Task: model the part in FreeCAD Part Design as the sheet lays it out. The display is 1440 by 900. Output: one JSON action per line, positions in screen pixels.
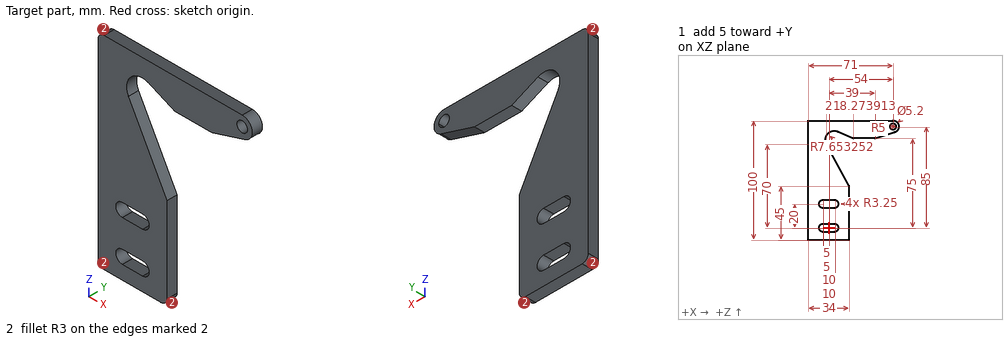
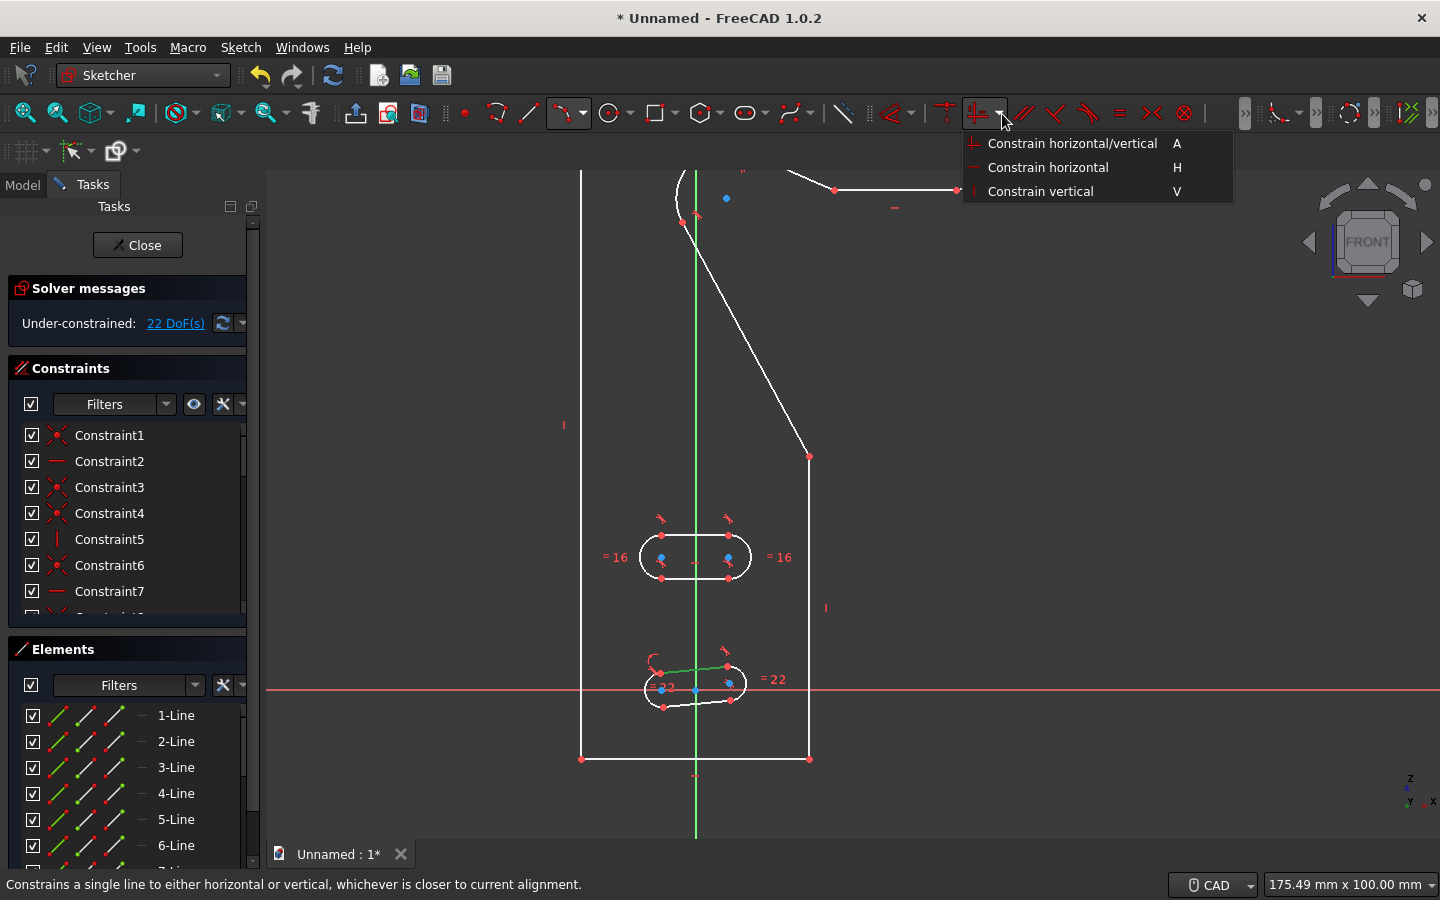
{"action": "left_click", "coordinate": [1098, 167]}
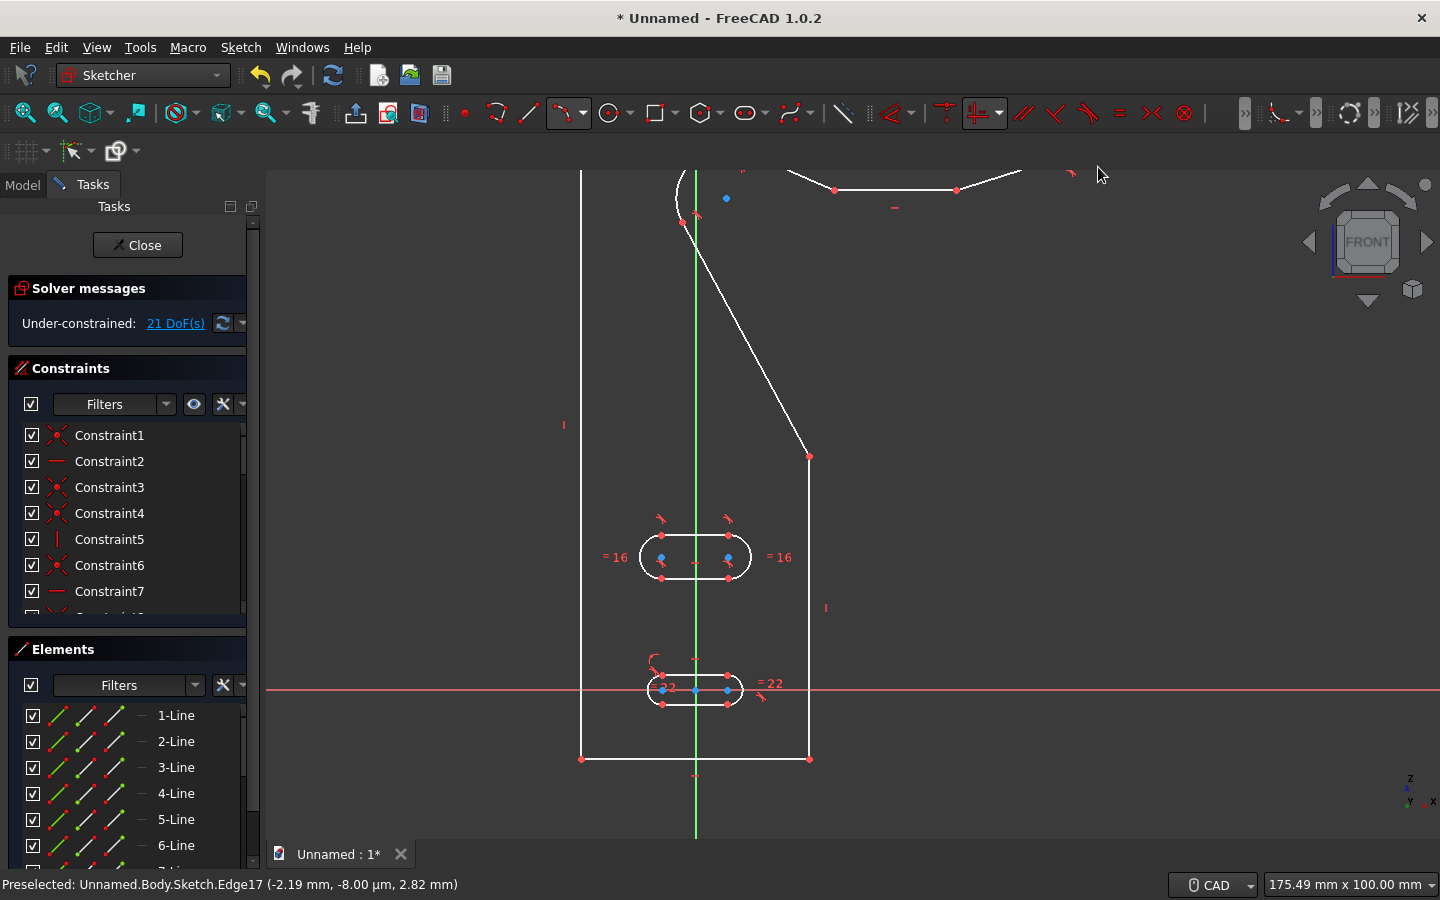
{"action": "left_click", "coordinate": [644, 544]}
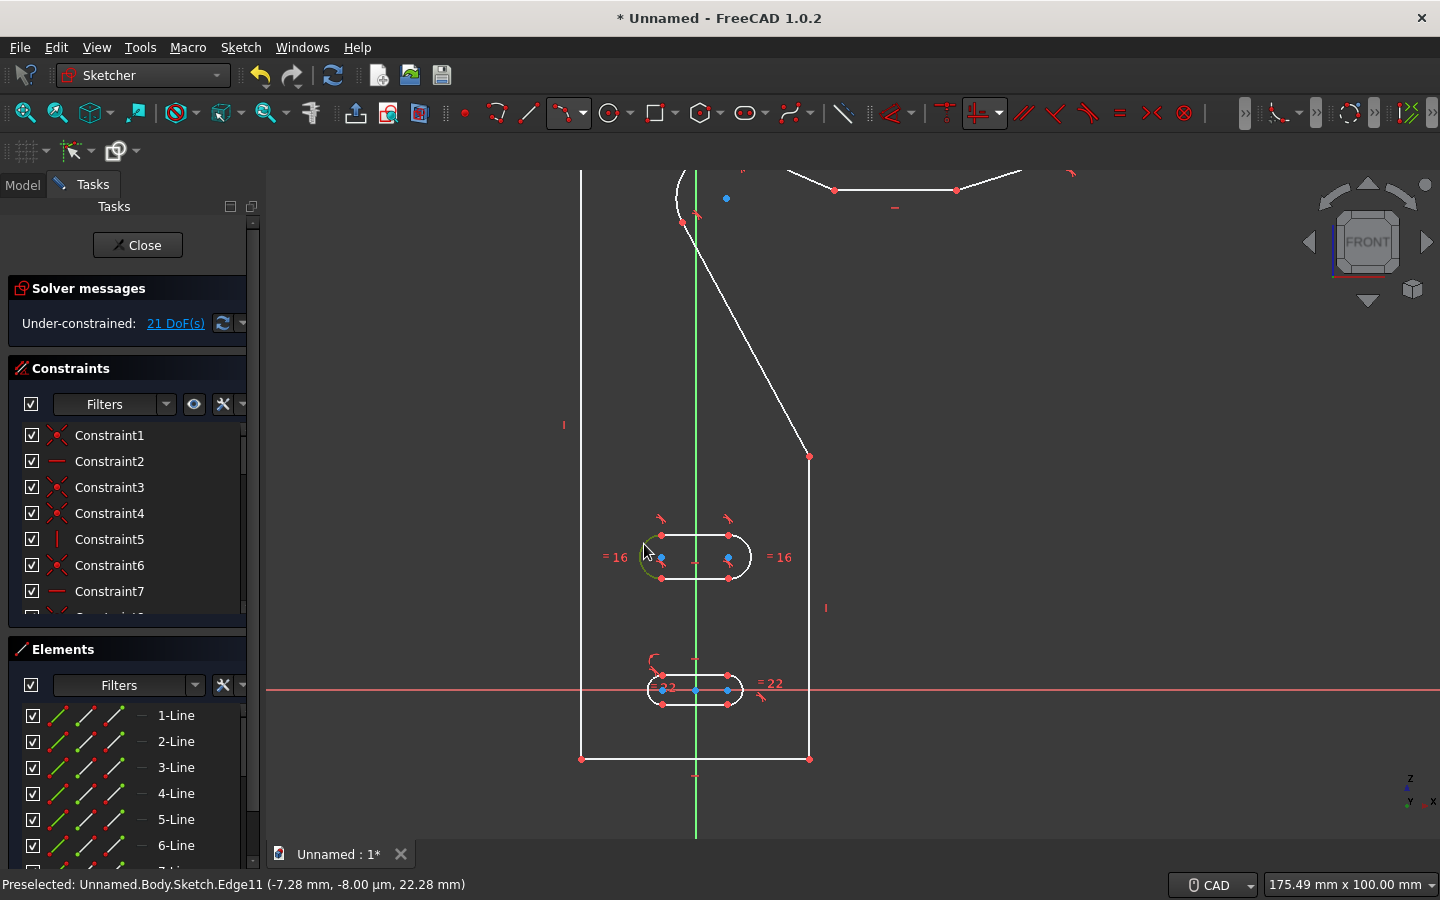
{"action": "left_click", "coordinate": [648, 690]}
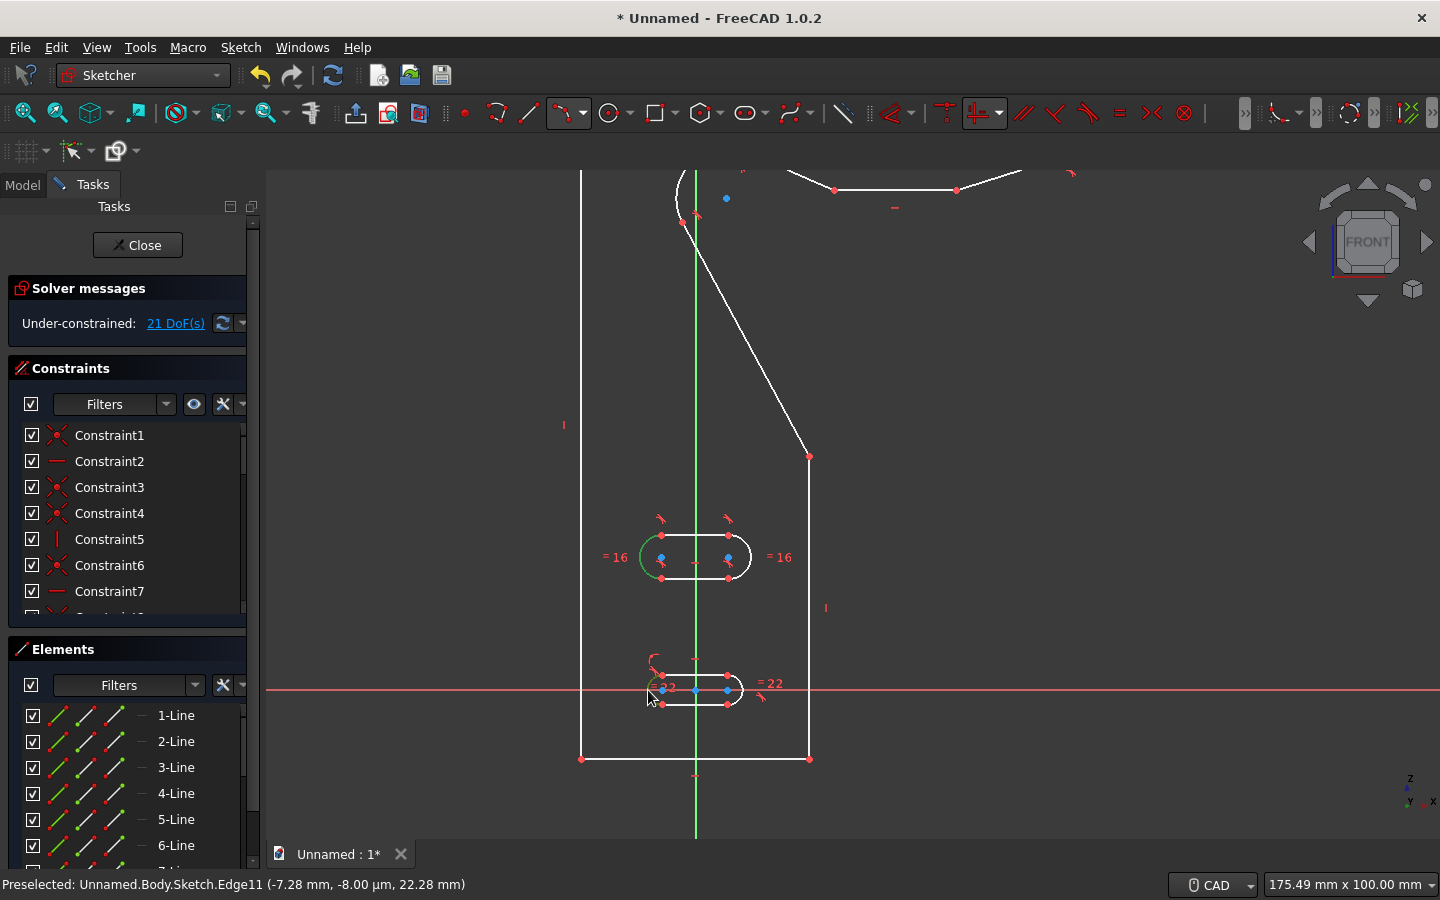
{"action": "left_click", "coordinate": [1120, 114]}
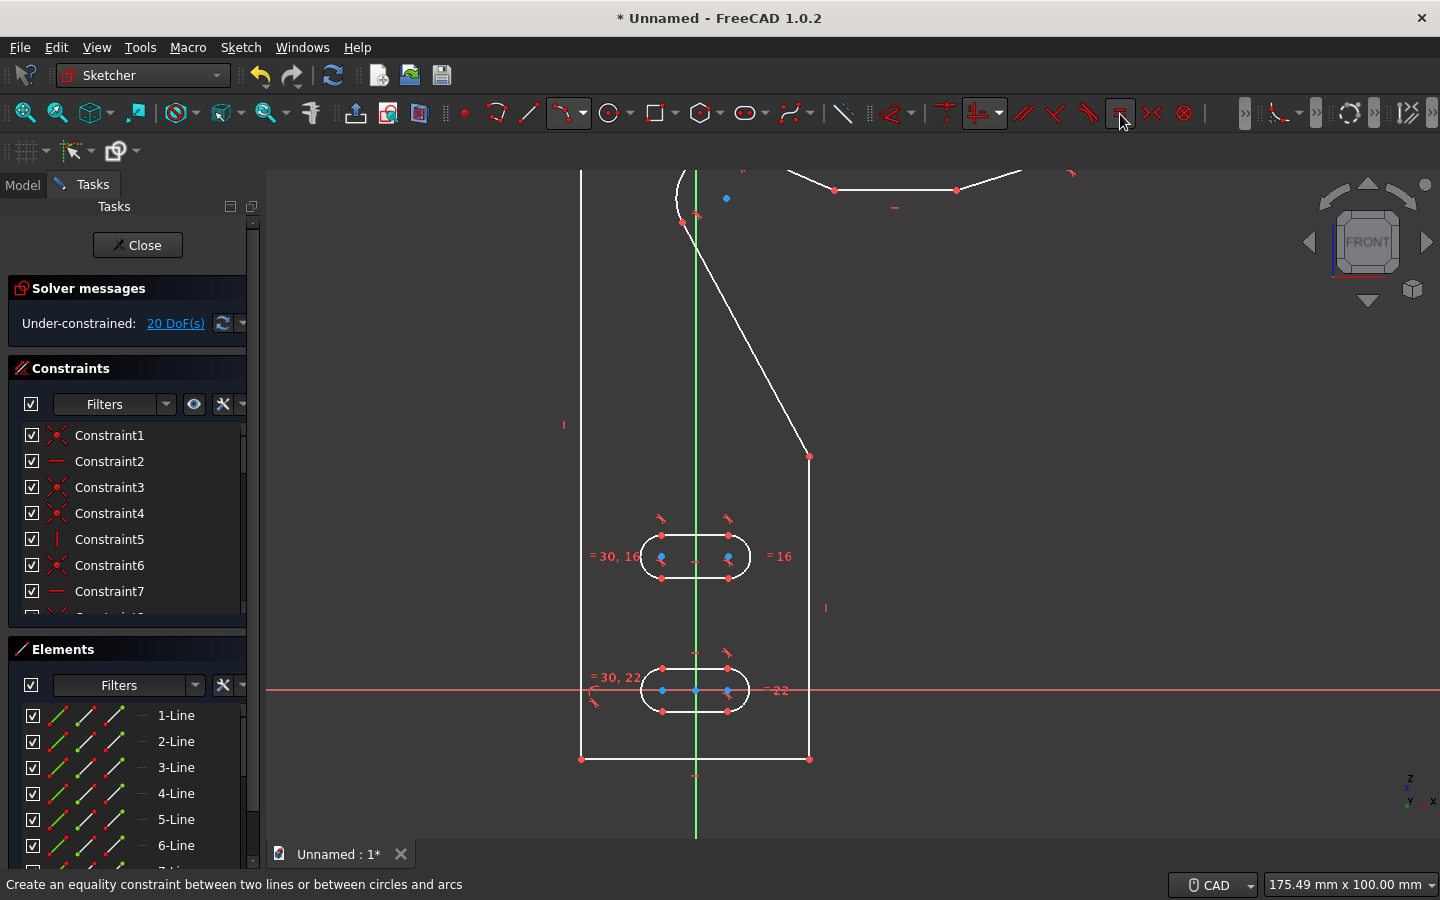
{"action": "key", "text": "d"}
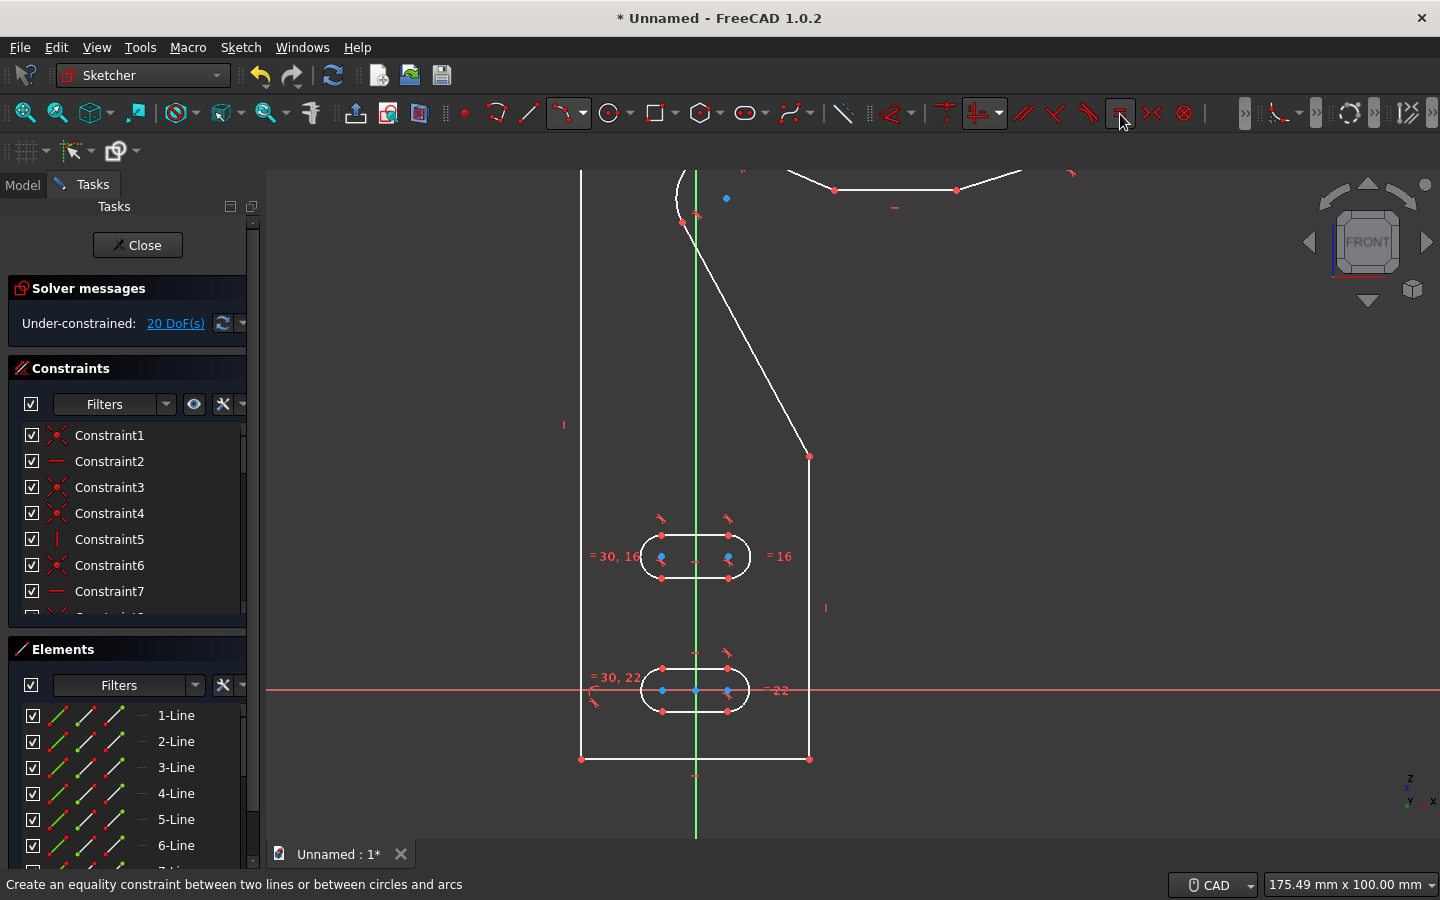
{"action": "left_click", "coordinate": [676, 199]}
{"action": "left_click", "coordinate": [644, 199]}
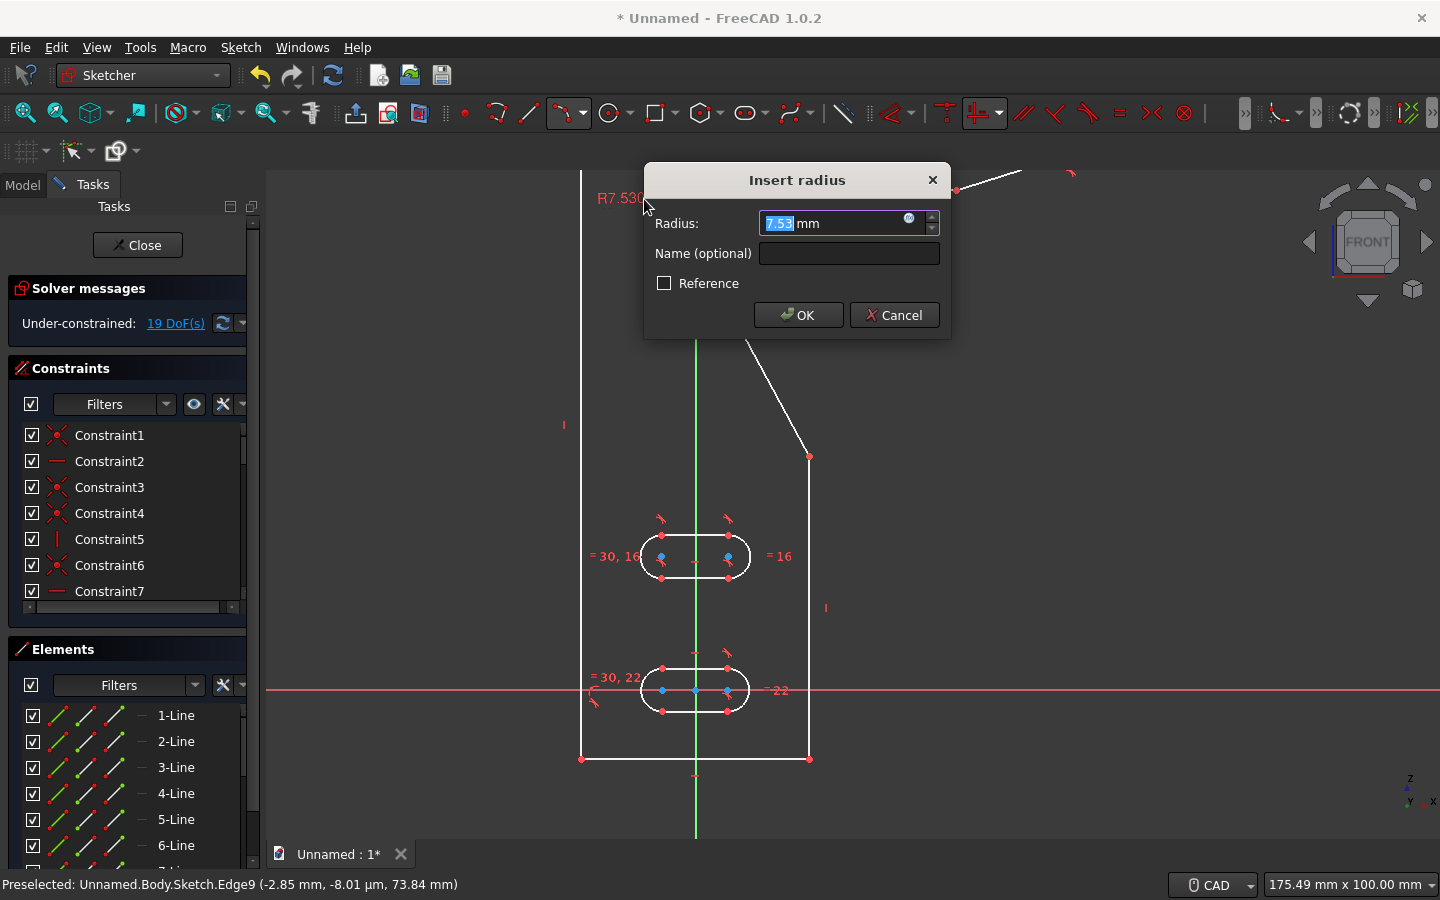
{"action": "type", "text": "7.653252"}
{"action": "key", "text": "Return"}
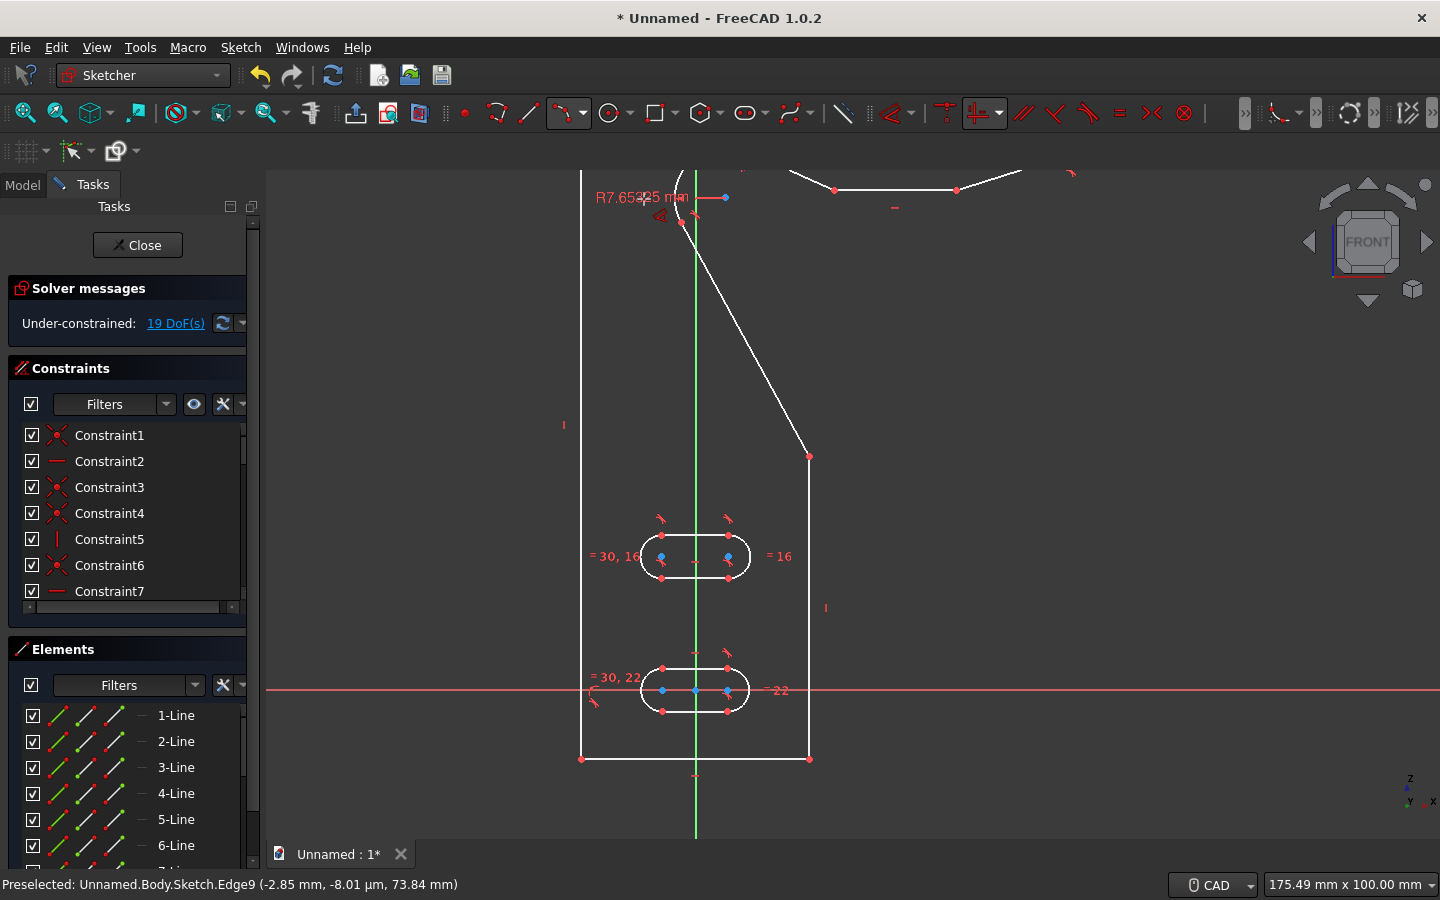
{"action": "scroll", "coordinate": [680, 671], "scroll_direction": "down", "scroll_amount": 2}